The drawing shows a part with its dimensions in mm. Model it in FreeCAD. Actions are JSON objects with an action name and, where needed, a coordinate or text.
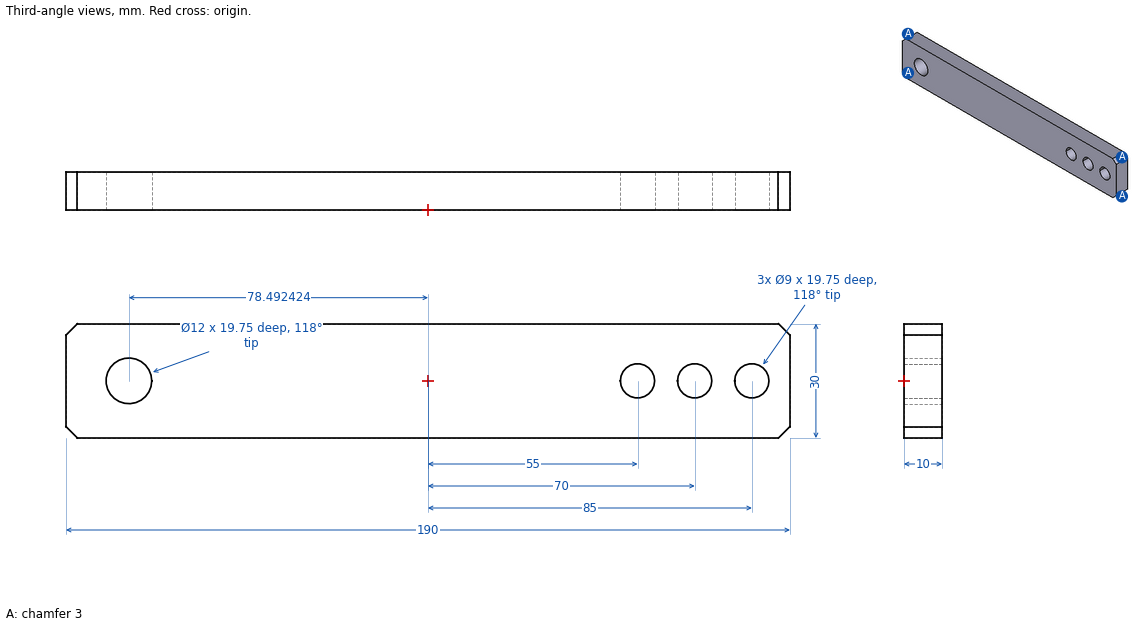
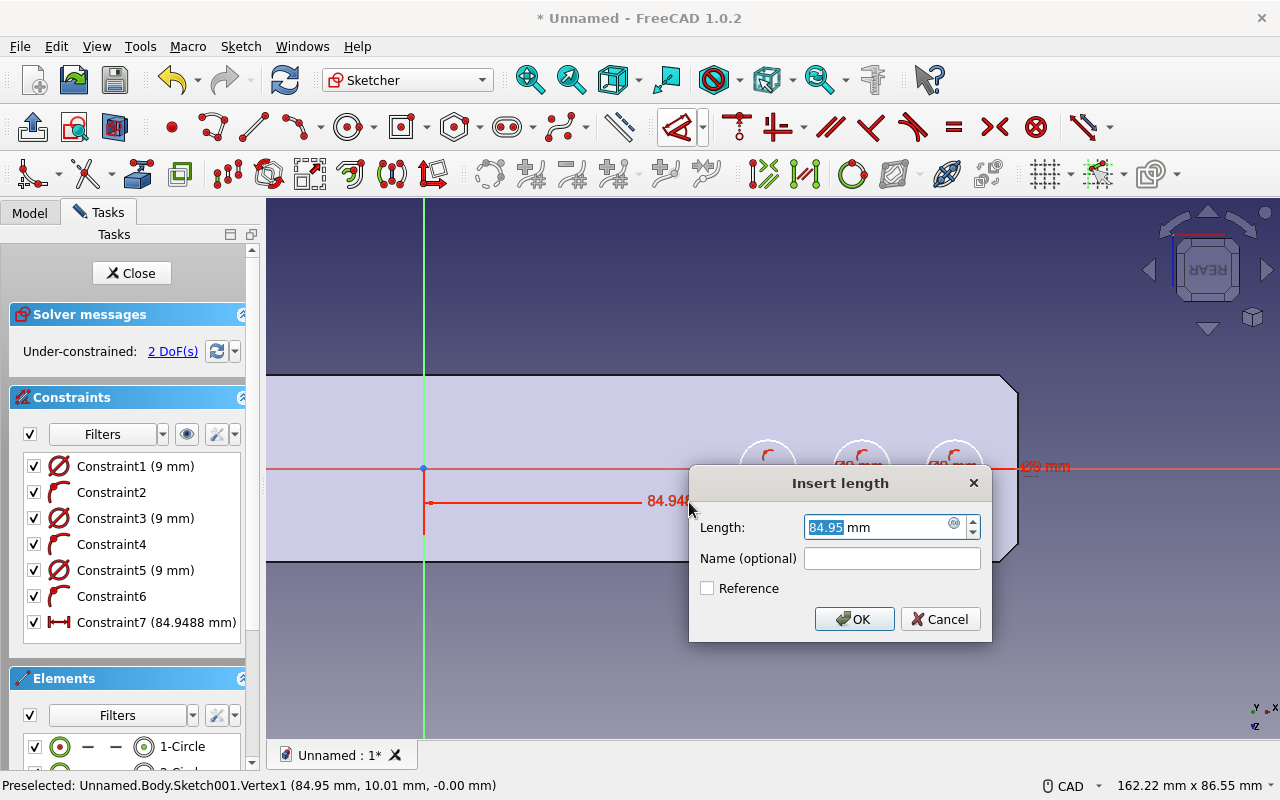
{"action": "type", "text": "85"}
{"action": "key", "text": "Return"}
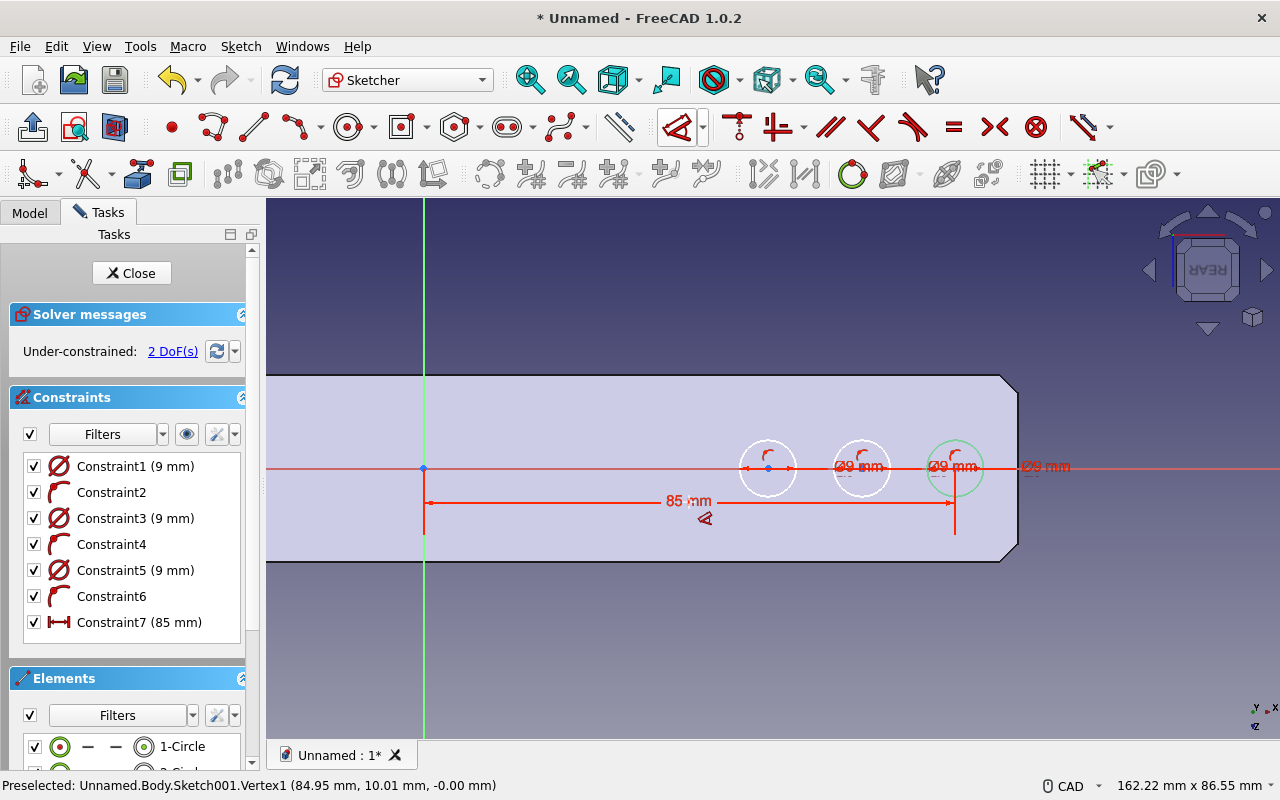
{"action": "left_click", "coordinate": [862, 468]}
{"action": "left_click", "coordinate": [542, 502]}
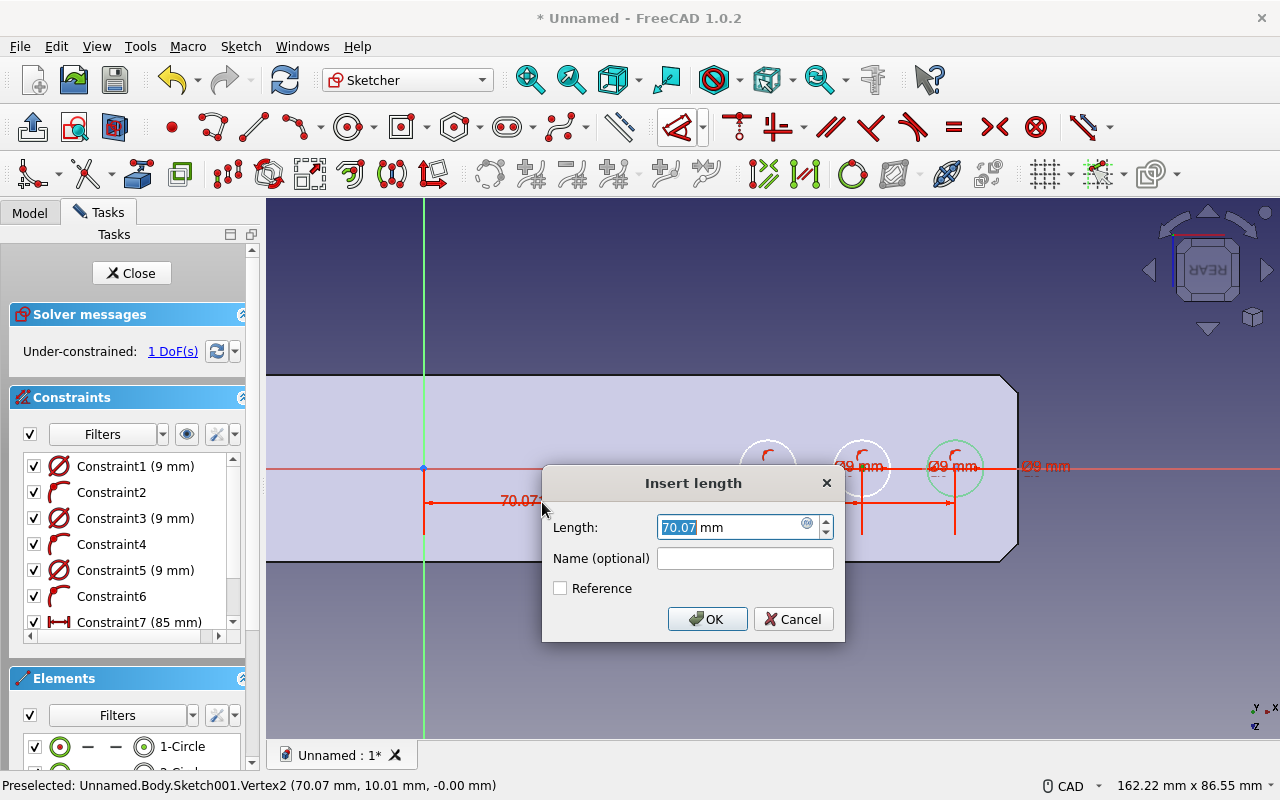
{"action": "type", "text": "70"}
{"action": "key", "text": "Return"}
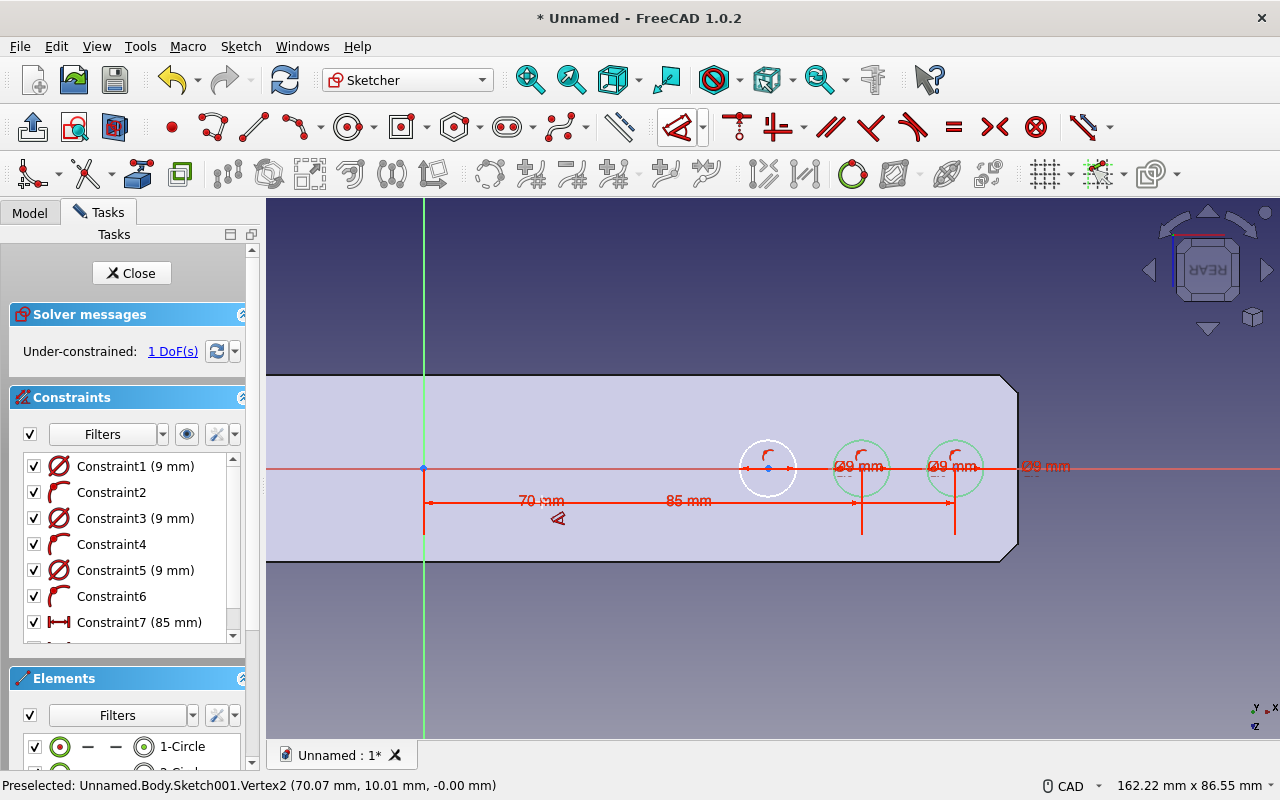
{"action": "left_click", "coordinate": [768, 468]}
{"action": "left_click", "coordinate": [596, 434]}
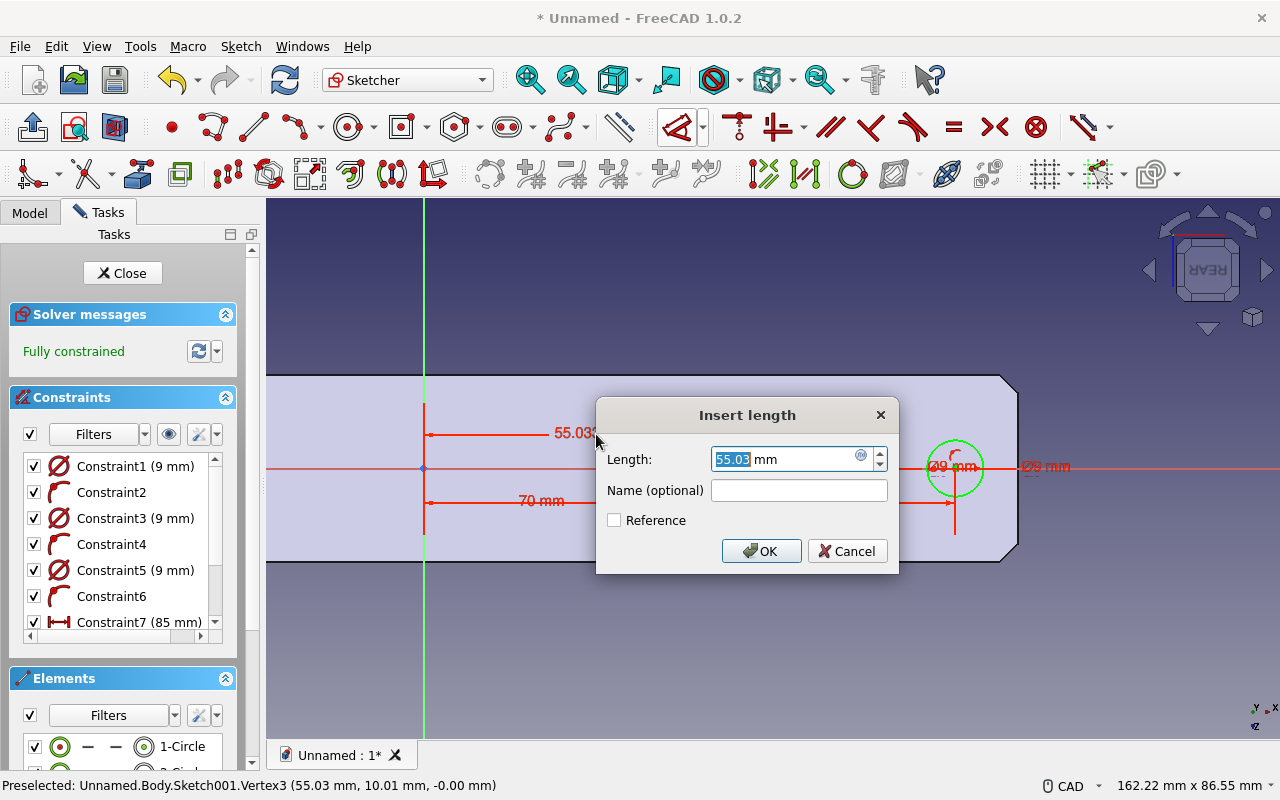
{"action": "type", "text": "55"}
{"action": "key", "text": "Return"}
{"action": "key", "text": "Escape"}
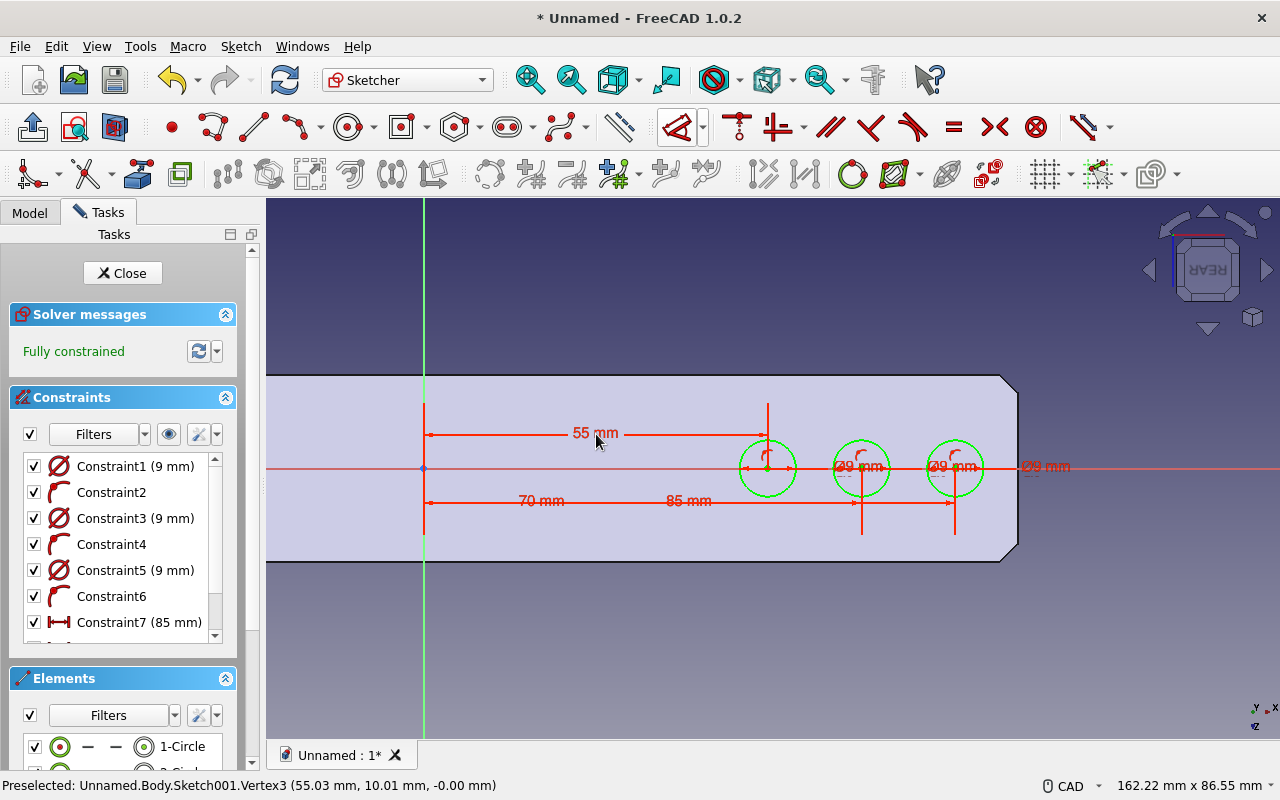
{"action": "left_click", "coordinate": [123, 273]}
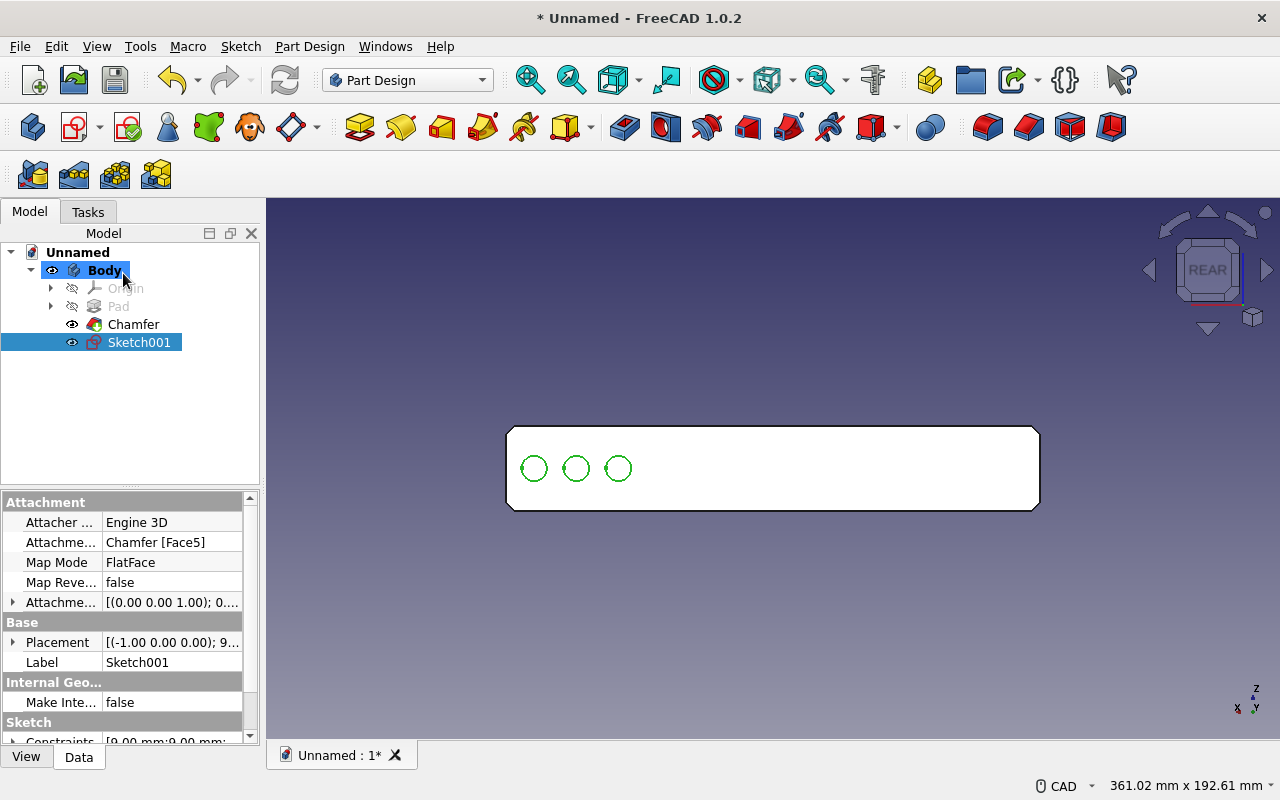
{"action": "left_click", "coordinate": [666, 128]}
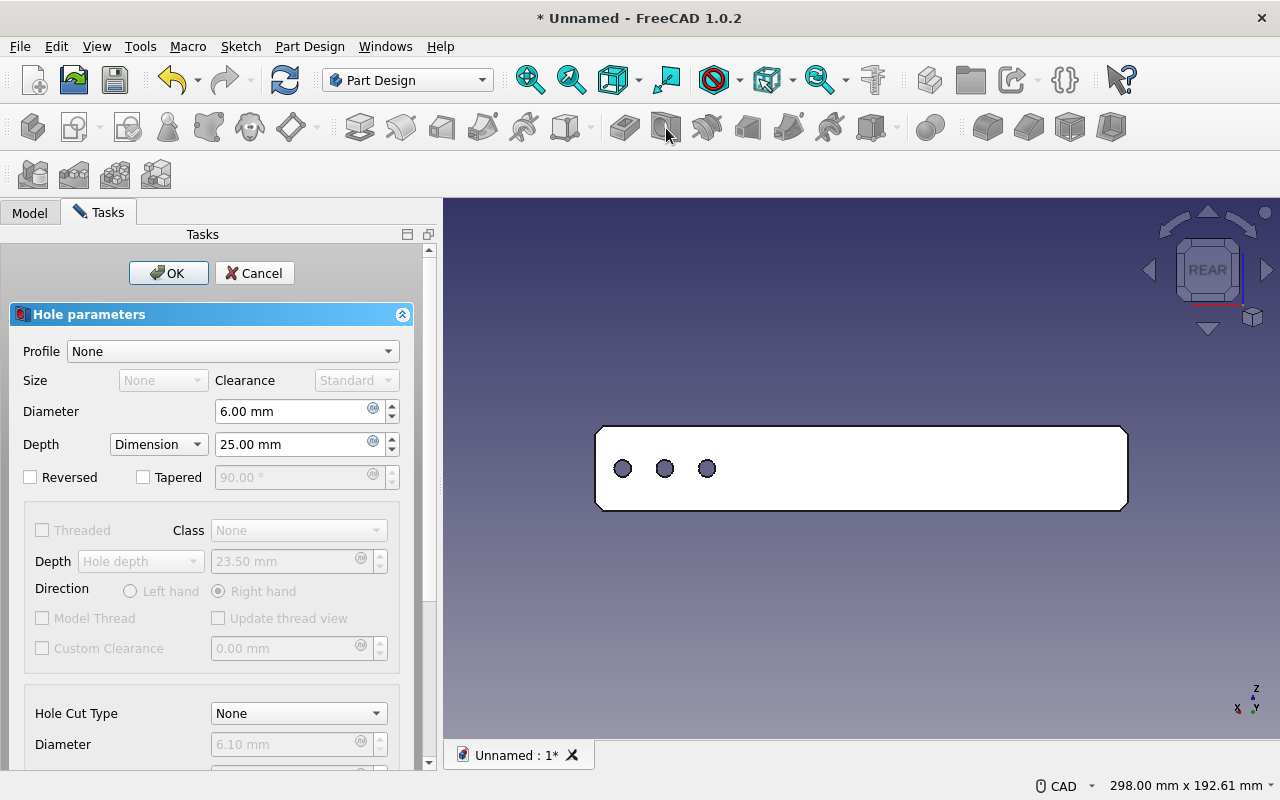
{"action": "triple_click", "coordinate": [300, 412]}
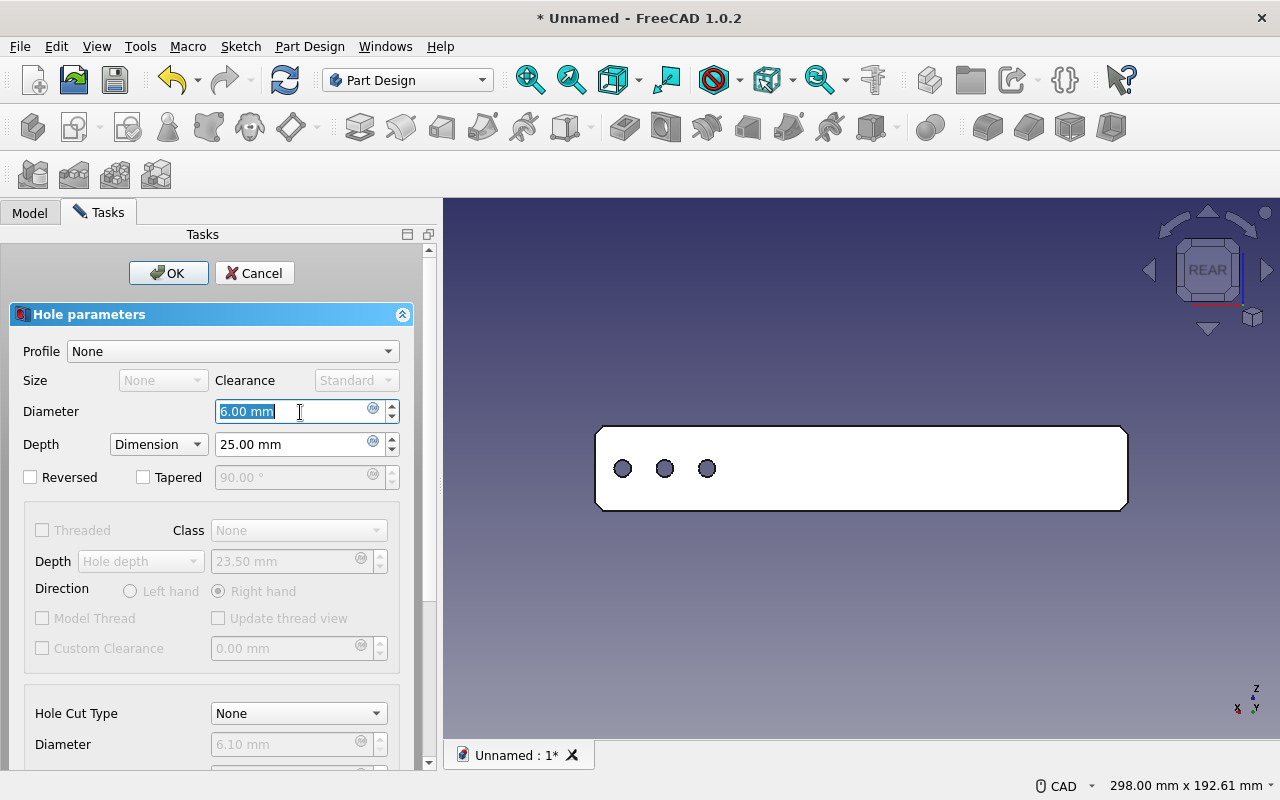
{"action": "type", "text": "9"}
{"action": "key", "text": "Tab"}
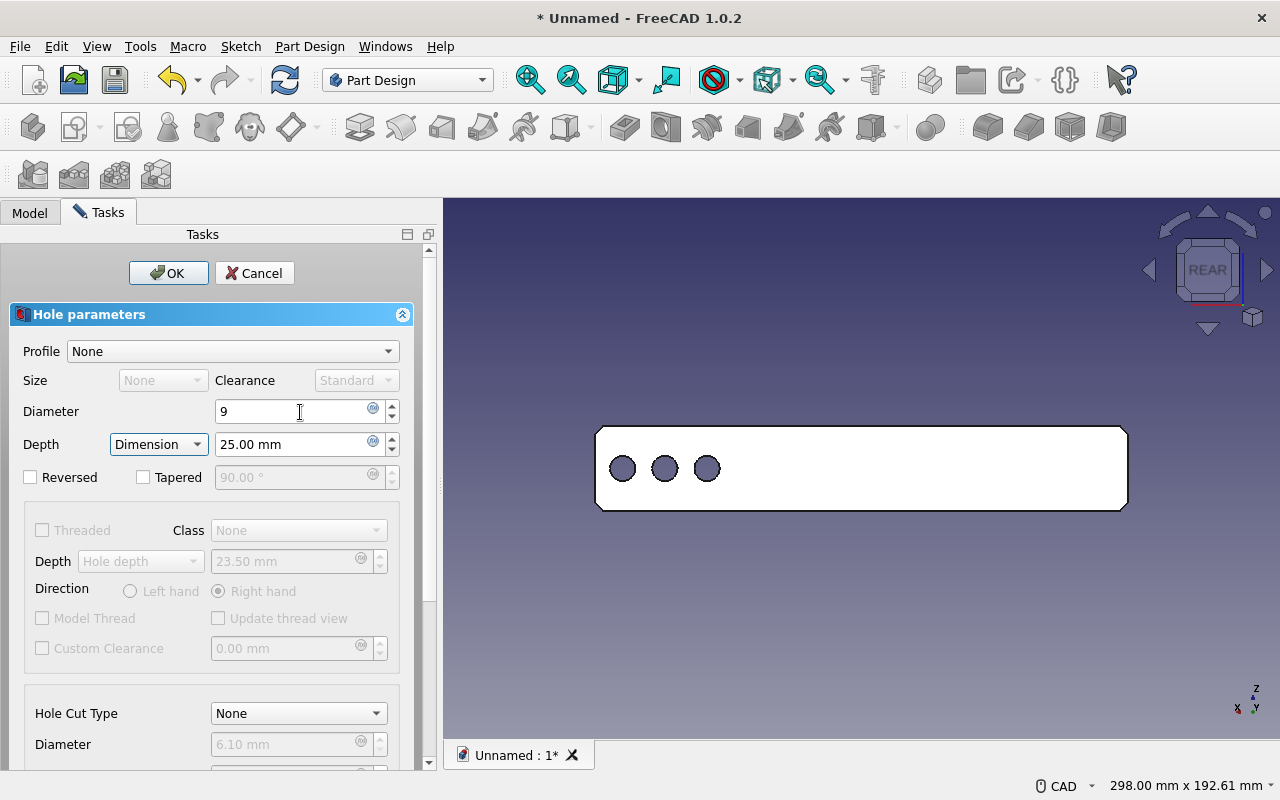
{"action": "triple_click", "coordinate": [300, 444]}